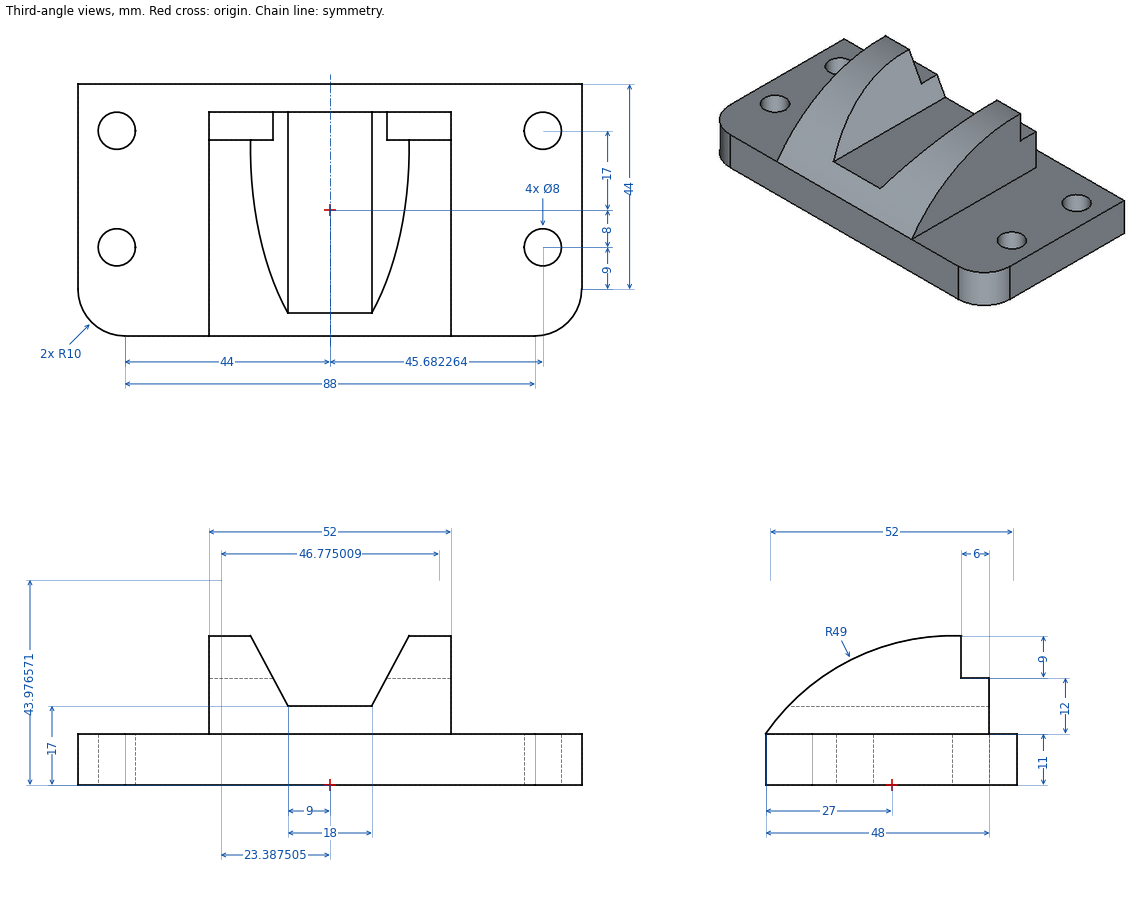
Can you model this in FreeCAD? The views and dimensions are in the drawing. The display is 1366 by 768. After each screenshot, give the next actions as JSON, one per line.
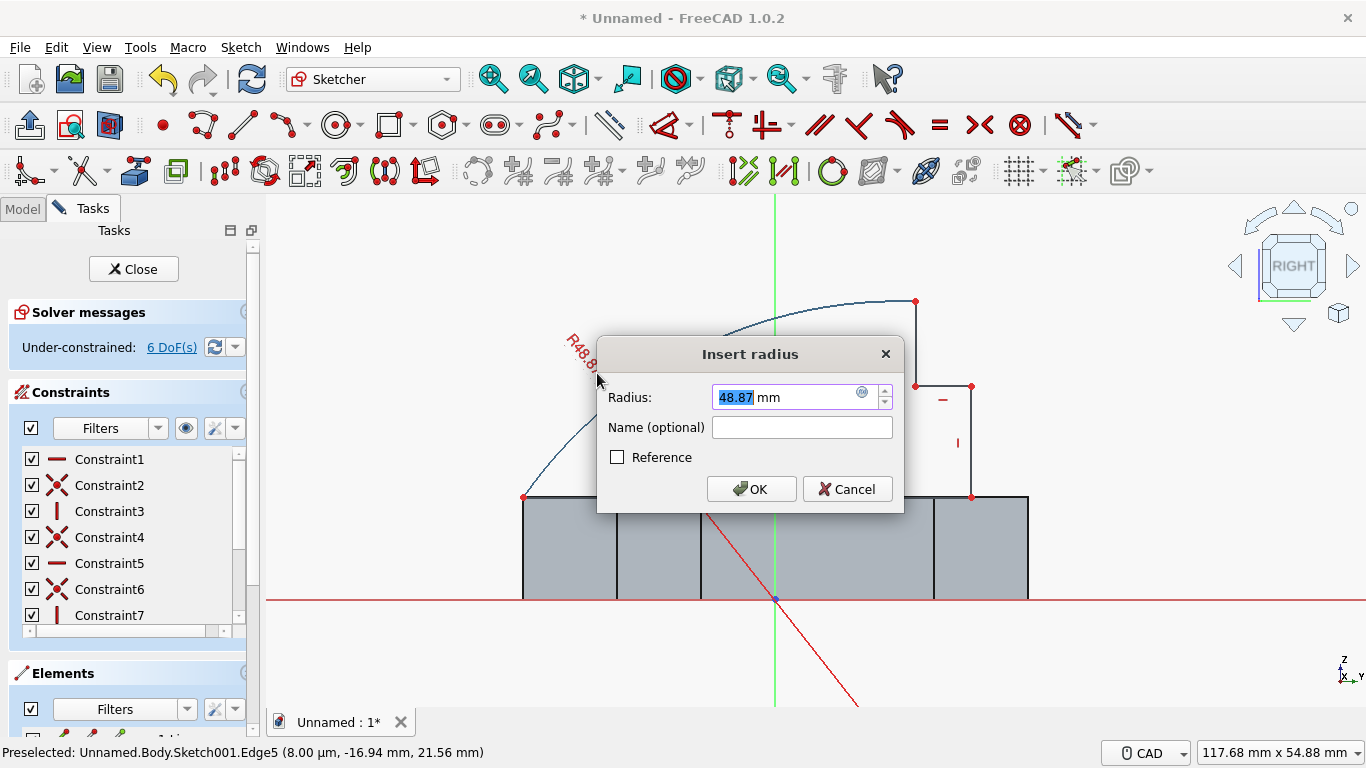
{"action": "type", "text": "49"}
{"action": "key", "text": "Return"}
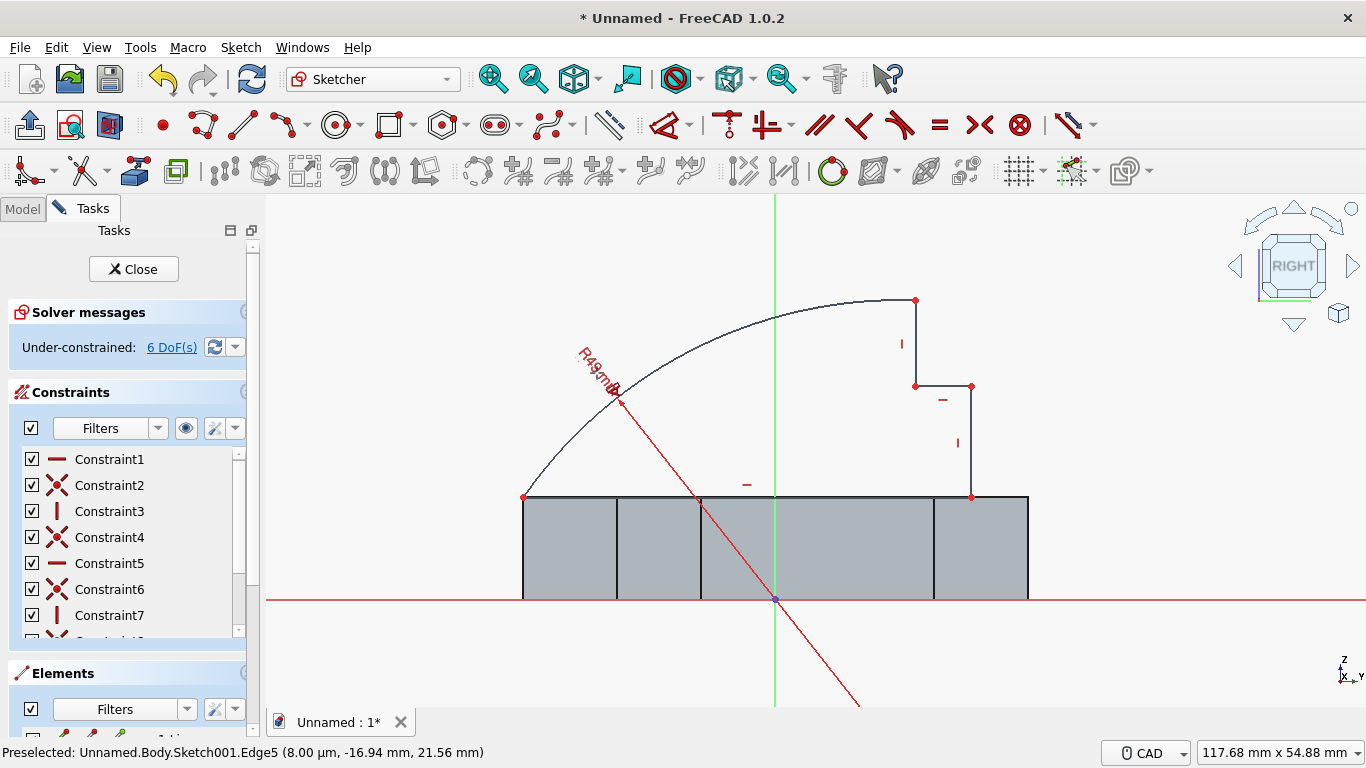
{"action": "left_click", "coordinate": [955, 386]}
{"action": "left_click", "coordinate": [944, 352]}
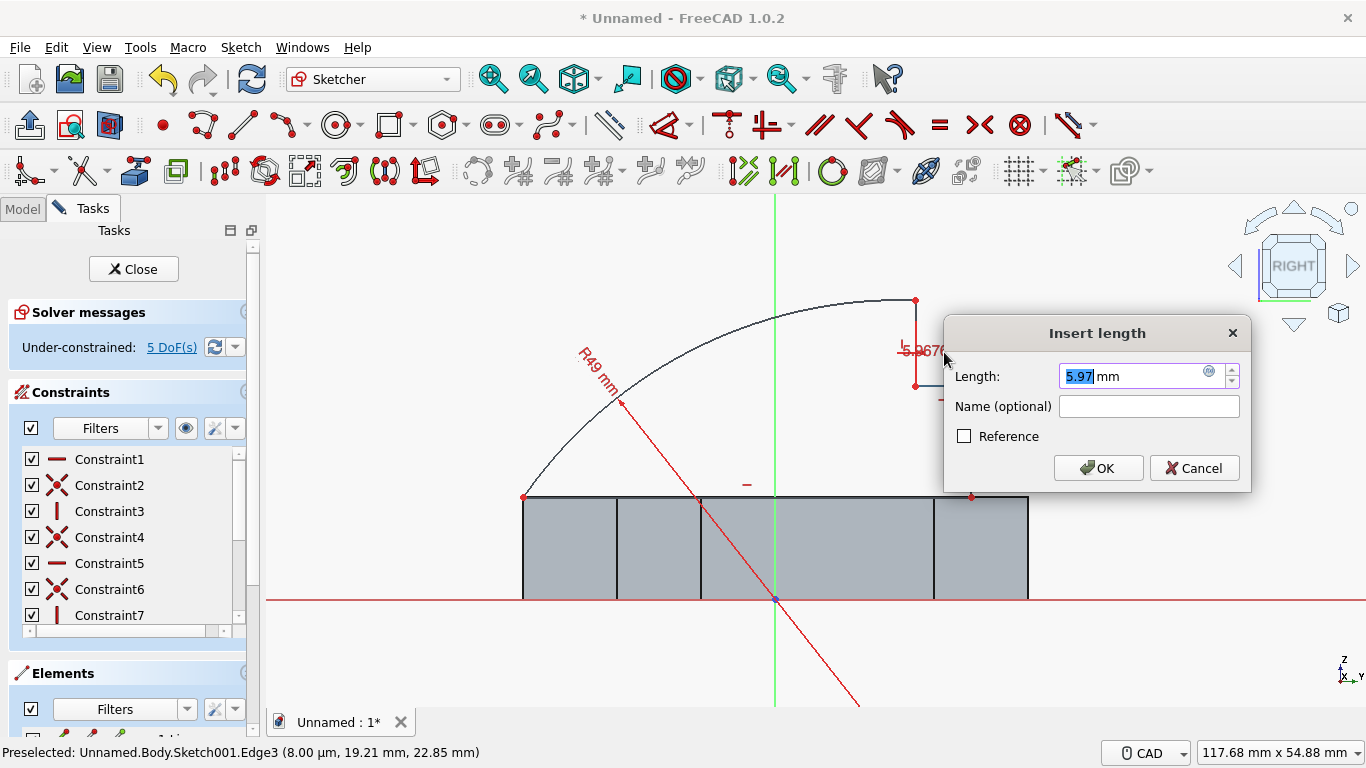
{"action": "type", "text": "6"}
{"action": "key", "text": "Return"}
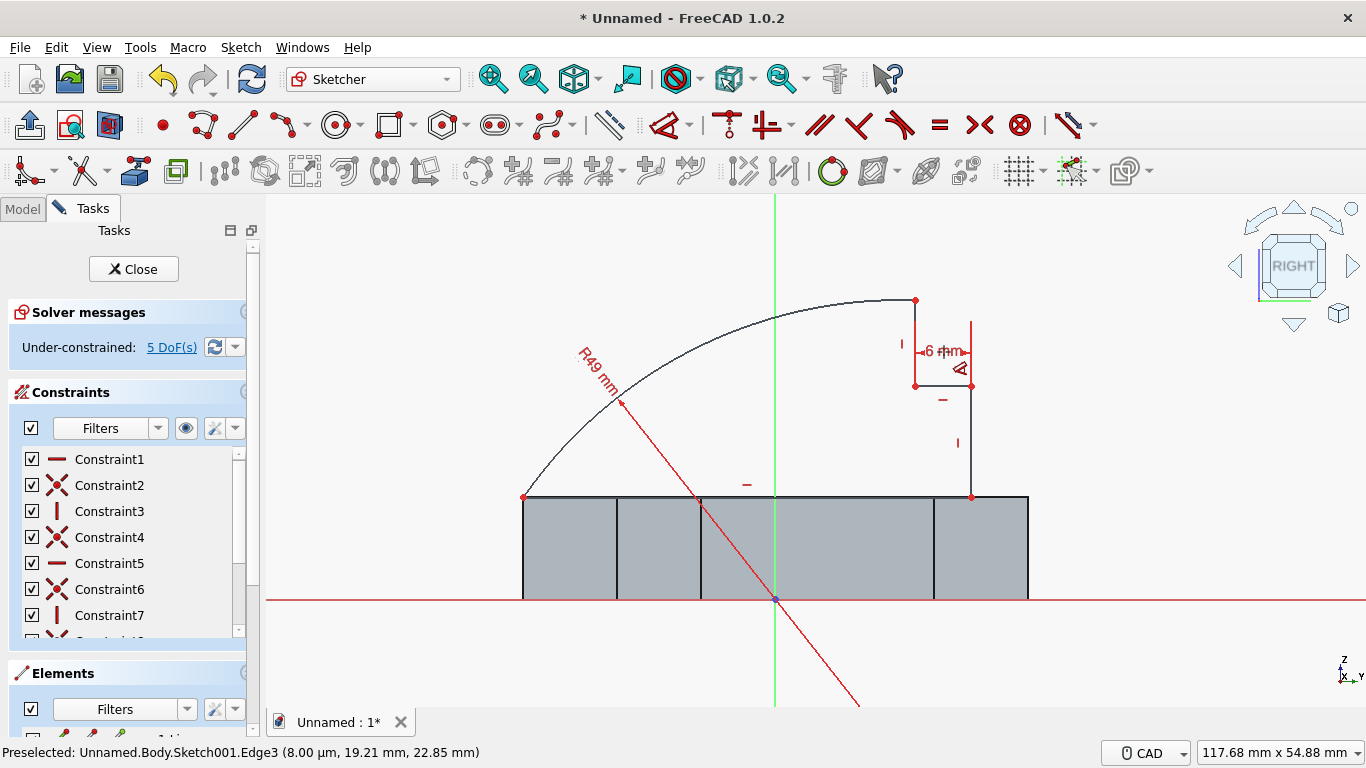
{"action": "left_click", "coordinate": [915, 360]}
{"action": "left_click", "coordinate": [949, 324]}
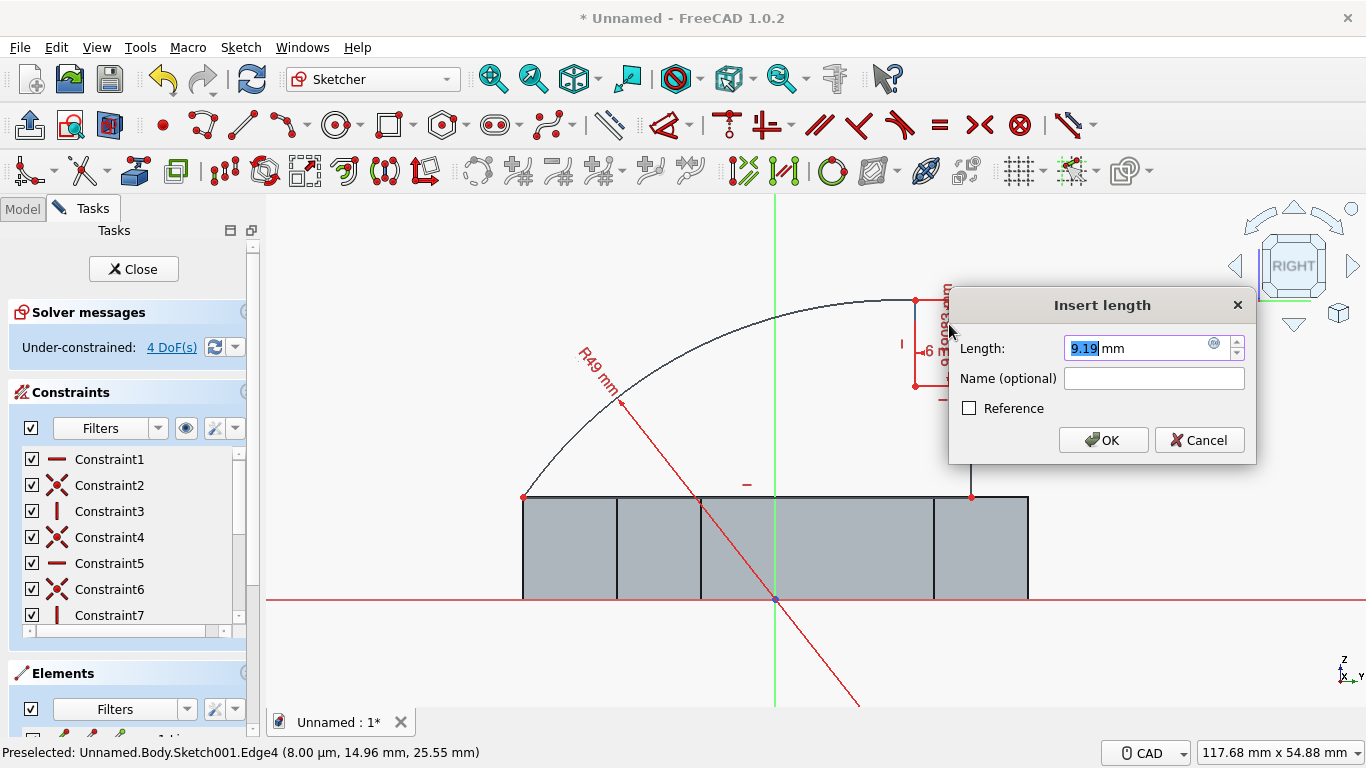
{"action": "type", "text": "9"}
{"action": "key", "text": "Return"}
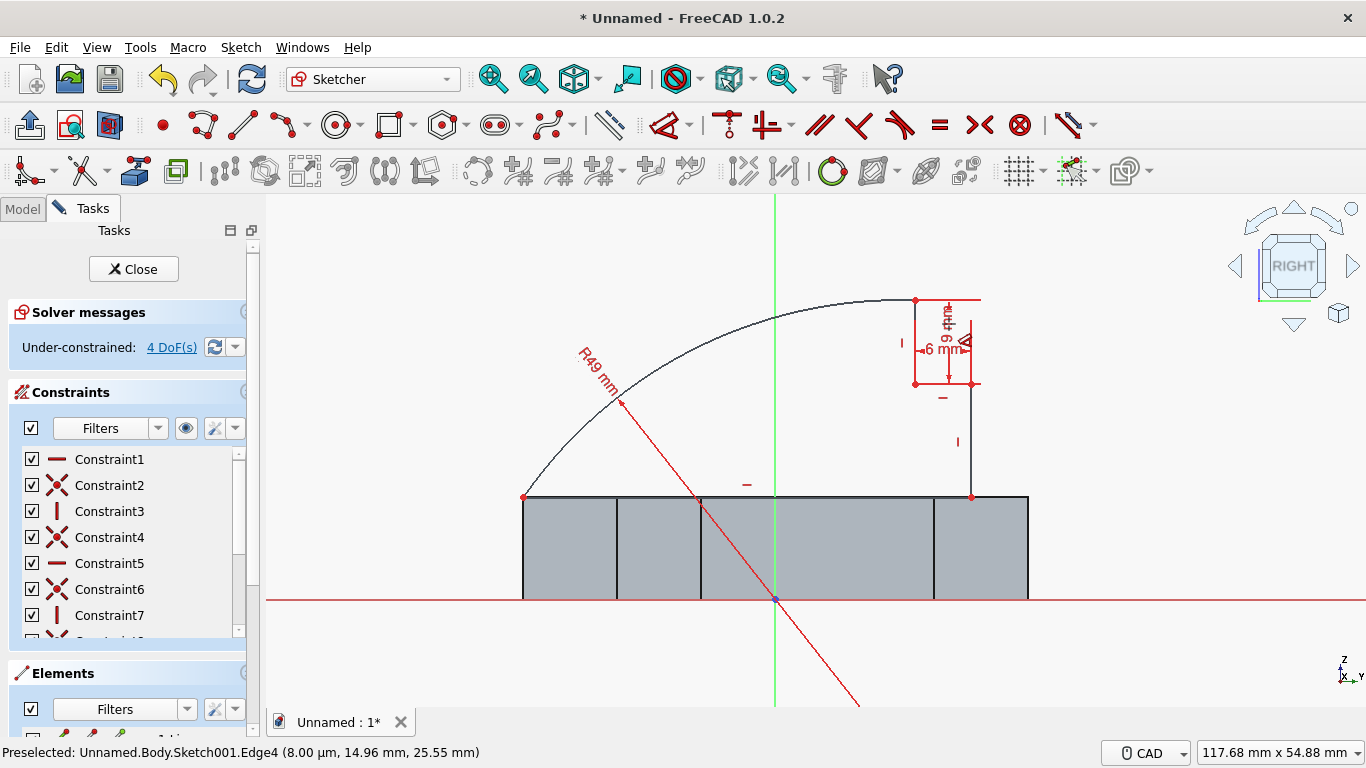
{"action": "left_click", "coordinate": [658, 498]}
{"action": "left_click", "coordinate": [747, 532]}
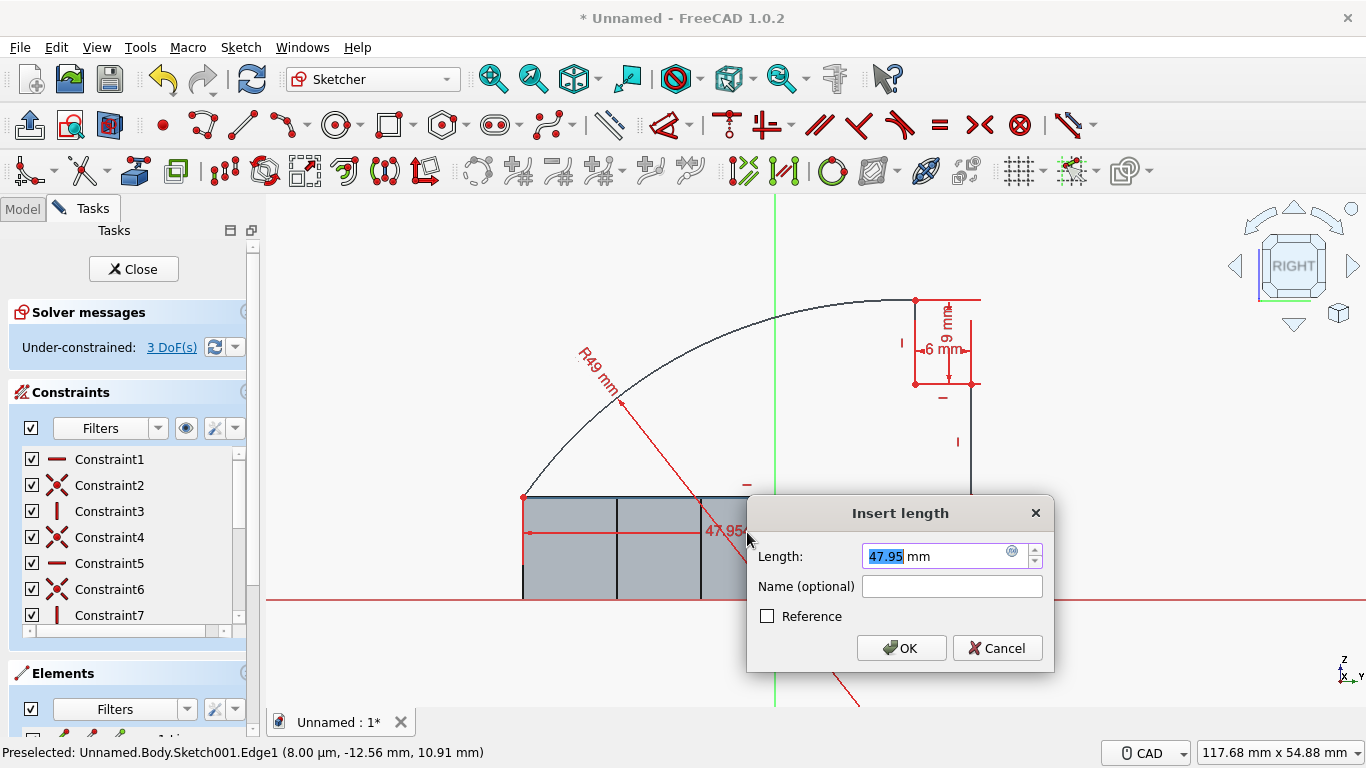
{"action": "type", "text": "48"}
{"action": "key", "text": "Return"}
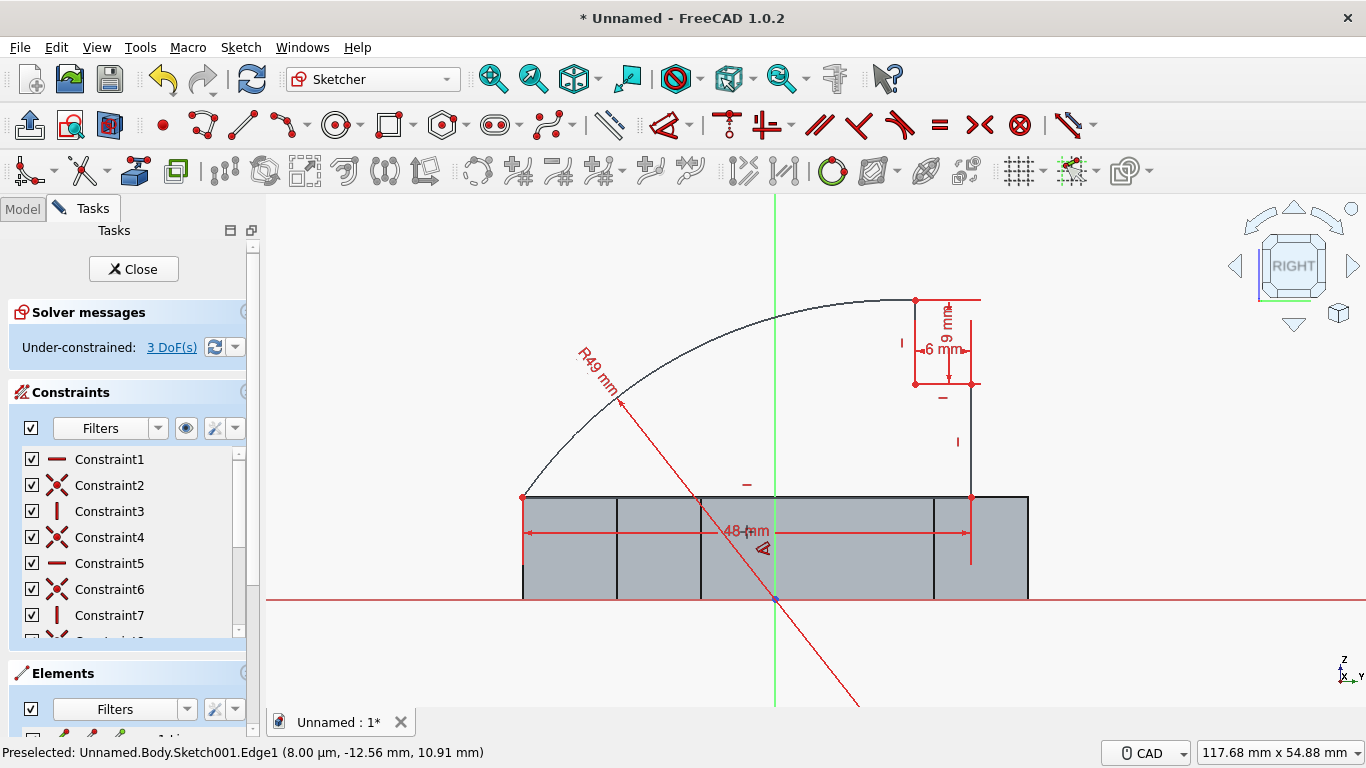
{"action": "left_click", "coordinate": [971, 464]}
{"action": "left_click", "coordinate": [1005, 441]}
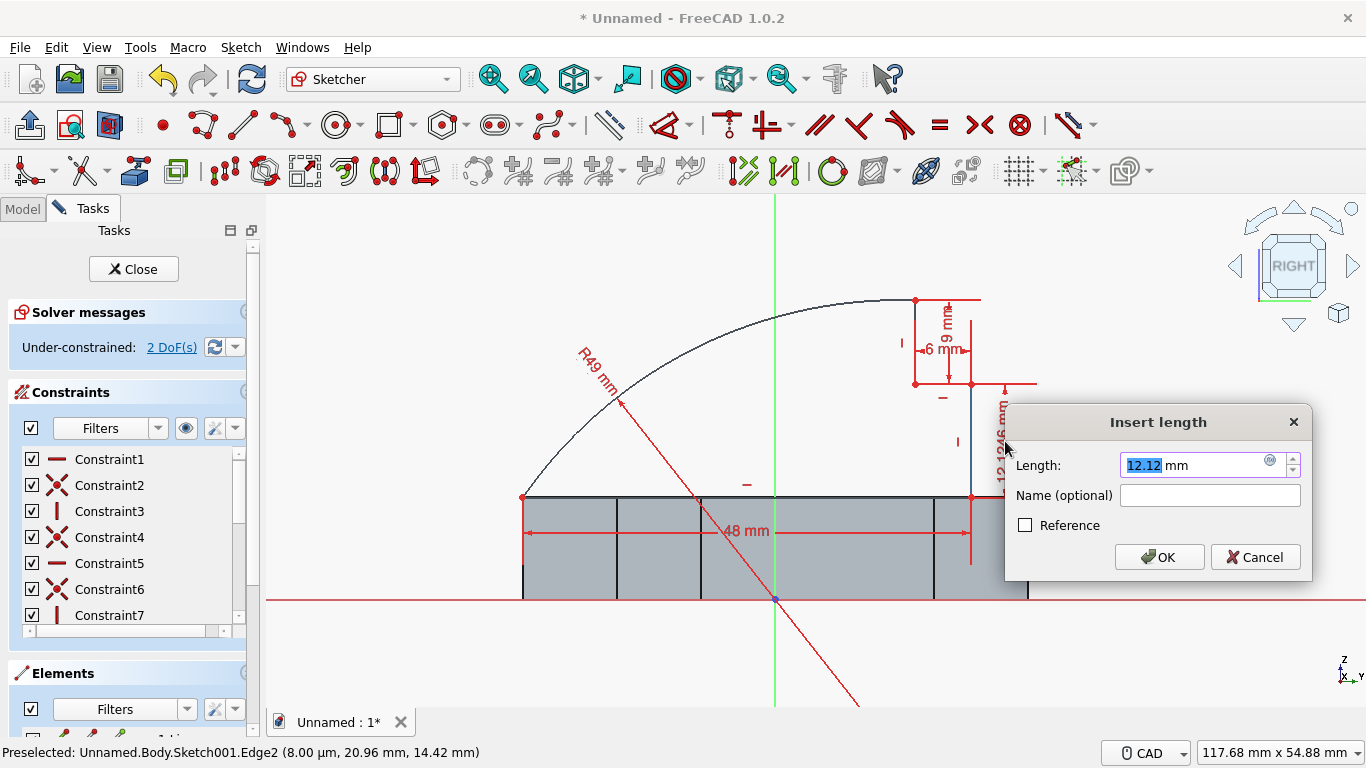
{"action": "type", "text": "12"}
{"action": "key", "text": "Return"}